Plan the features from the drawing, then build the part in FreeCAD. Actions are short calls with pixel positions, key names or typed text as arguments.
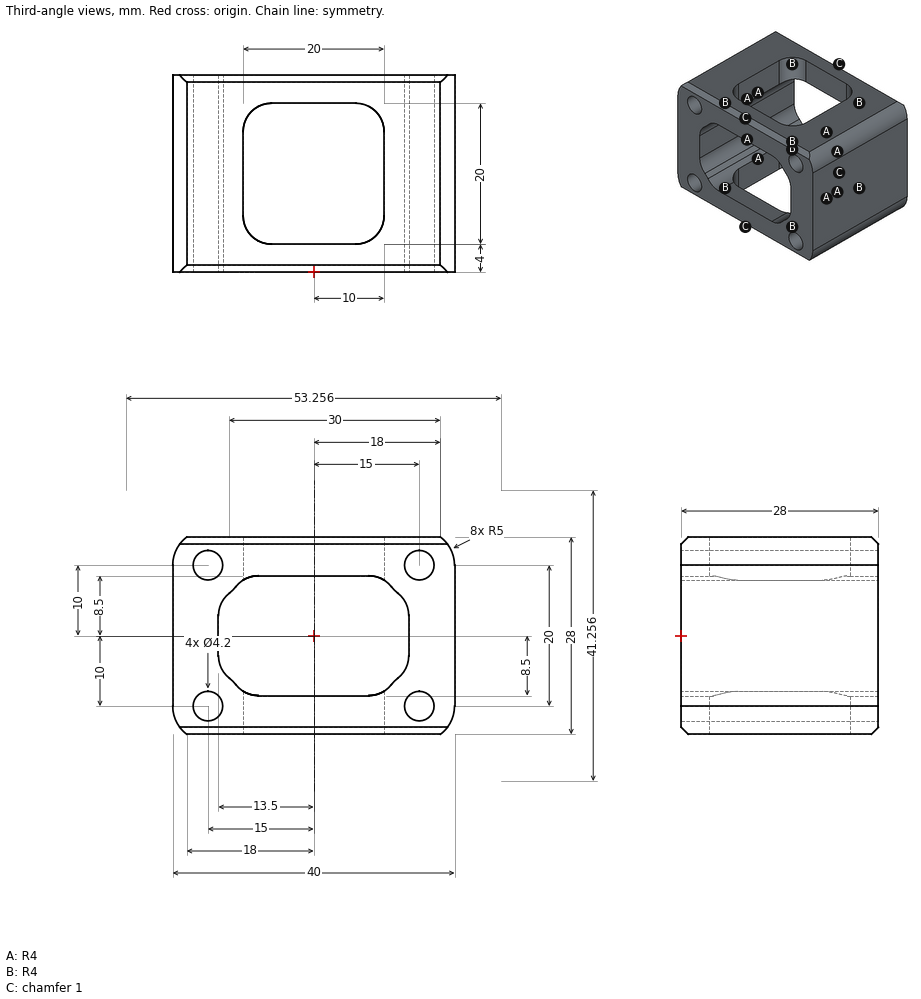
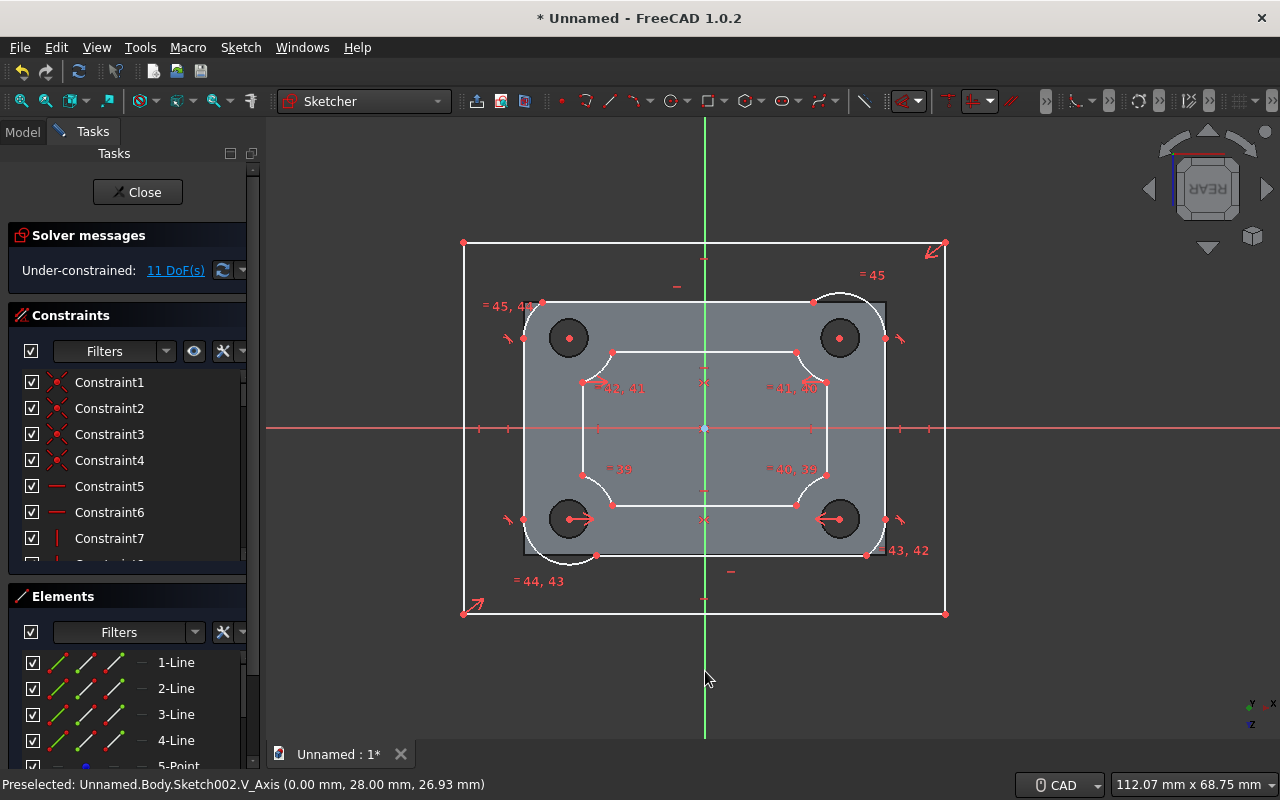
click(607, 494)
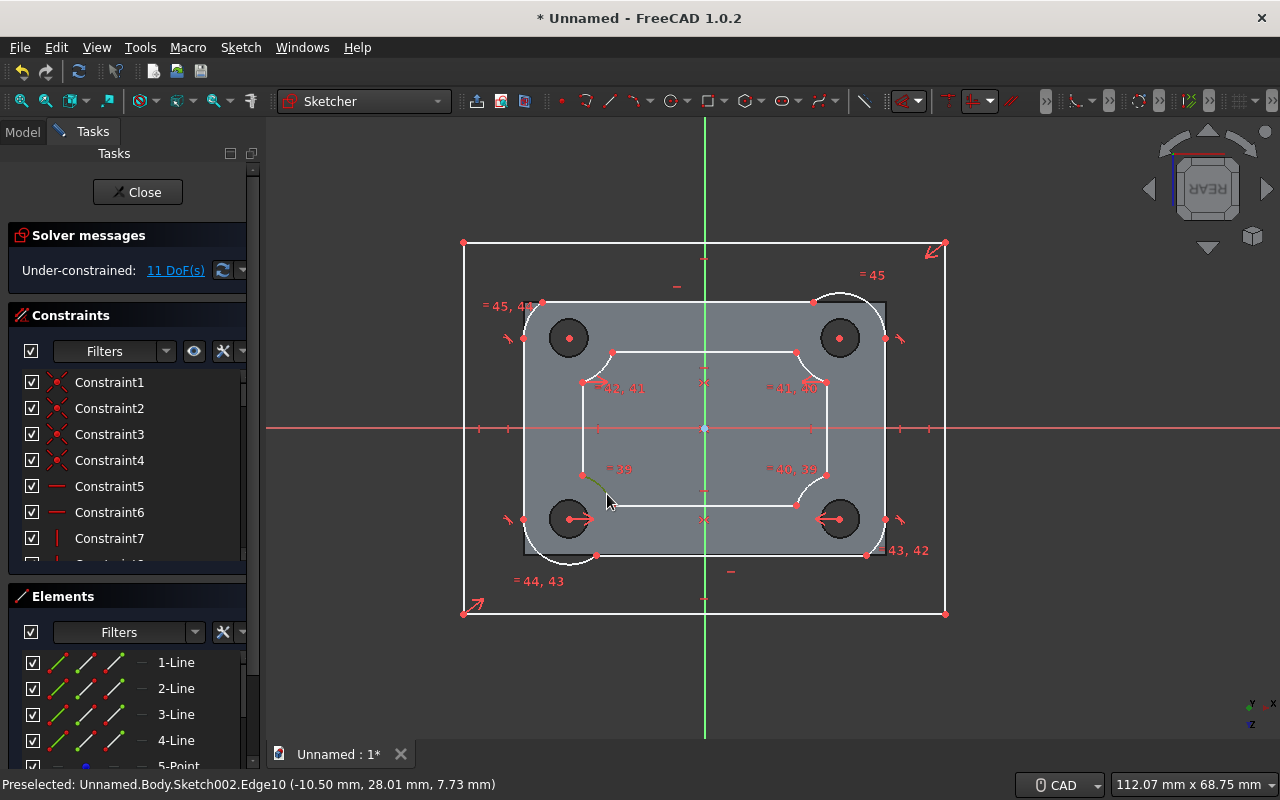
click(920, 102)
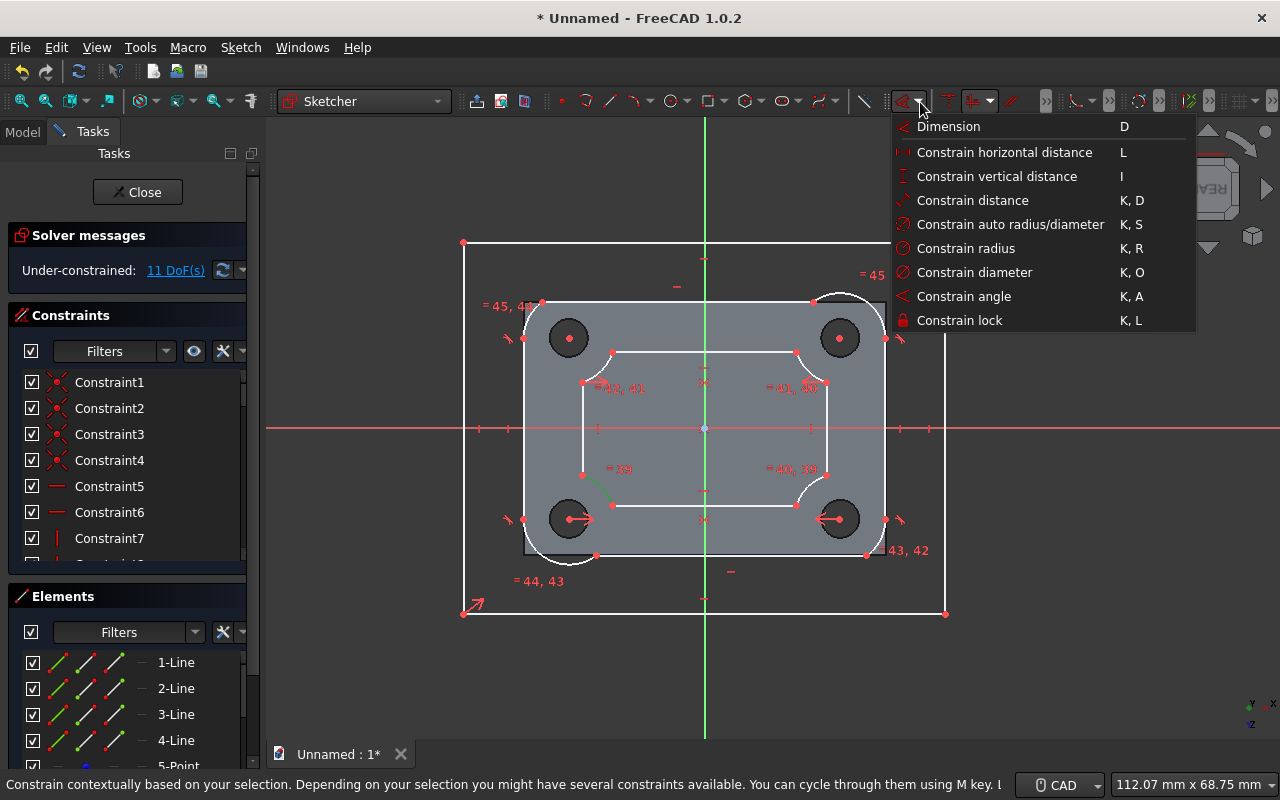
click(1044, 248)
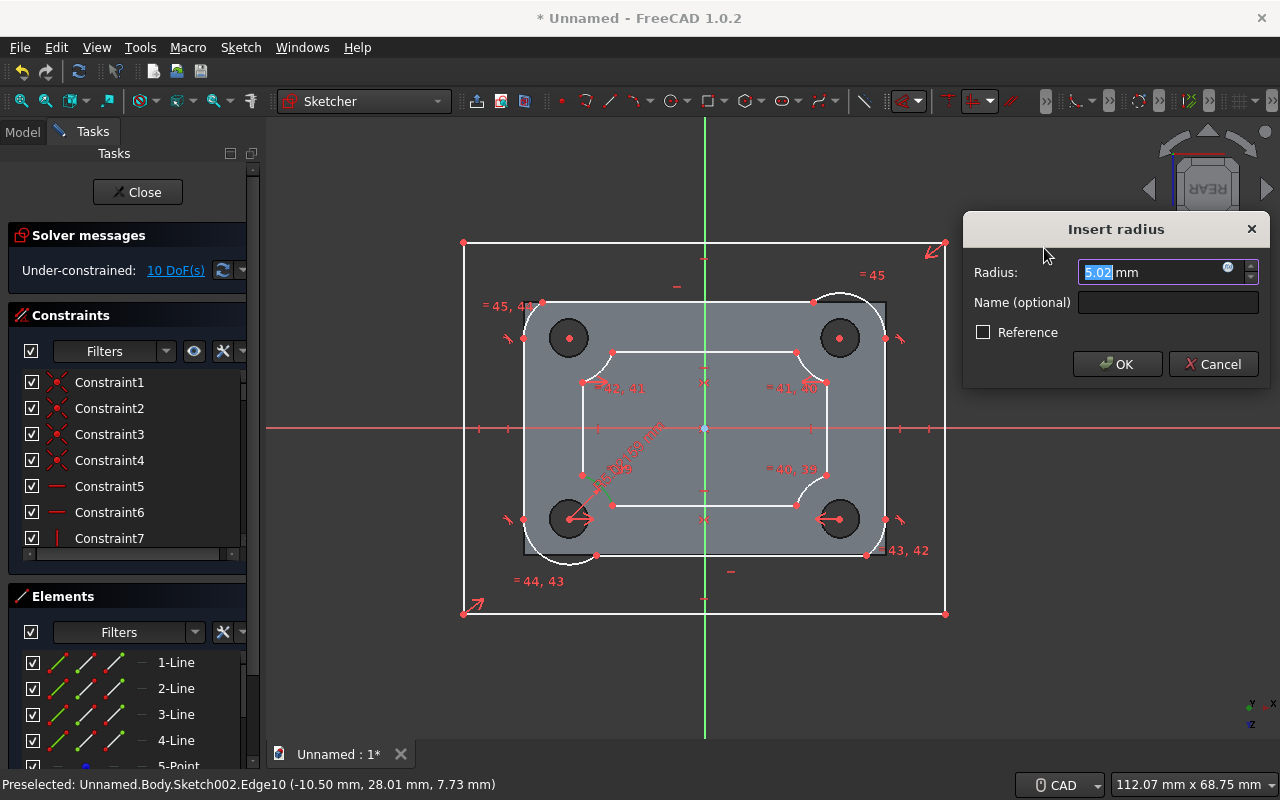
text(5)
key(Return)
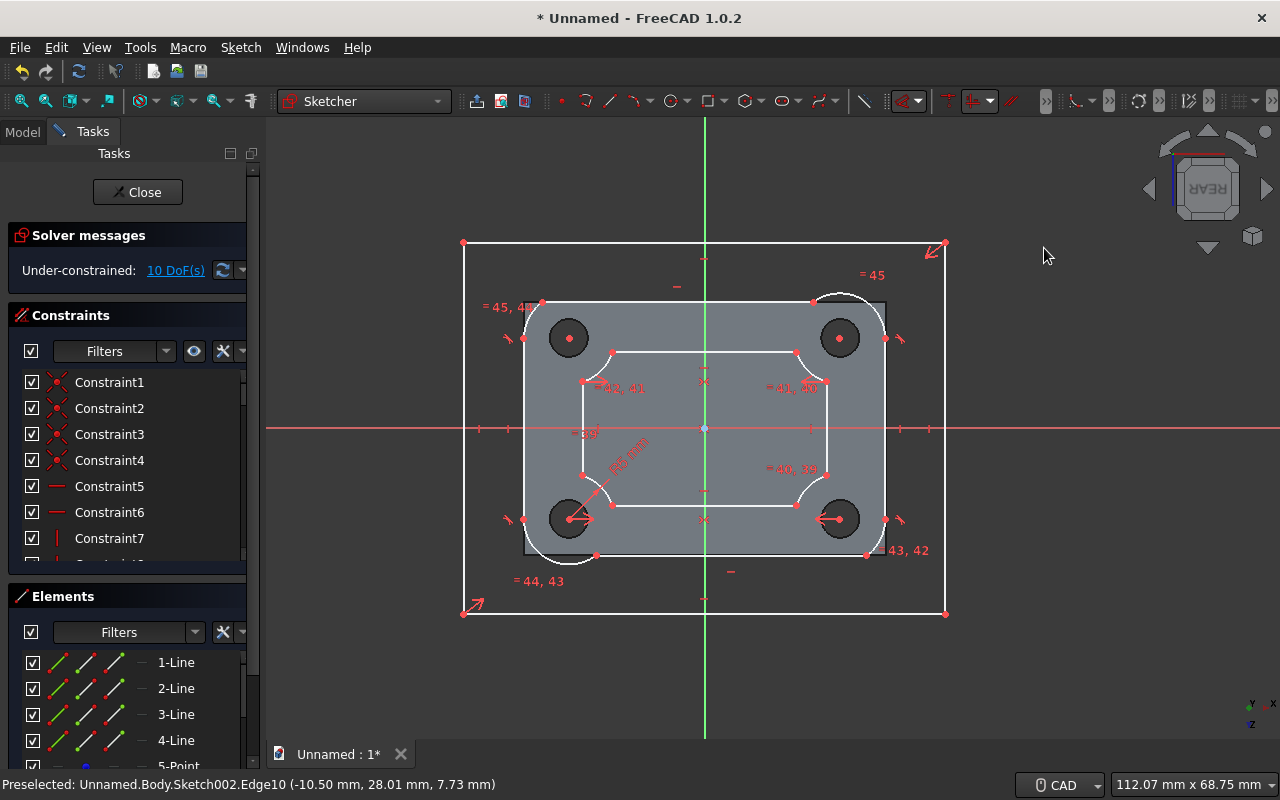
click(885, 393)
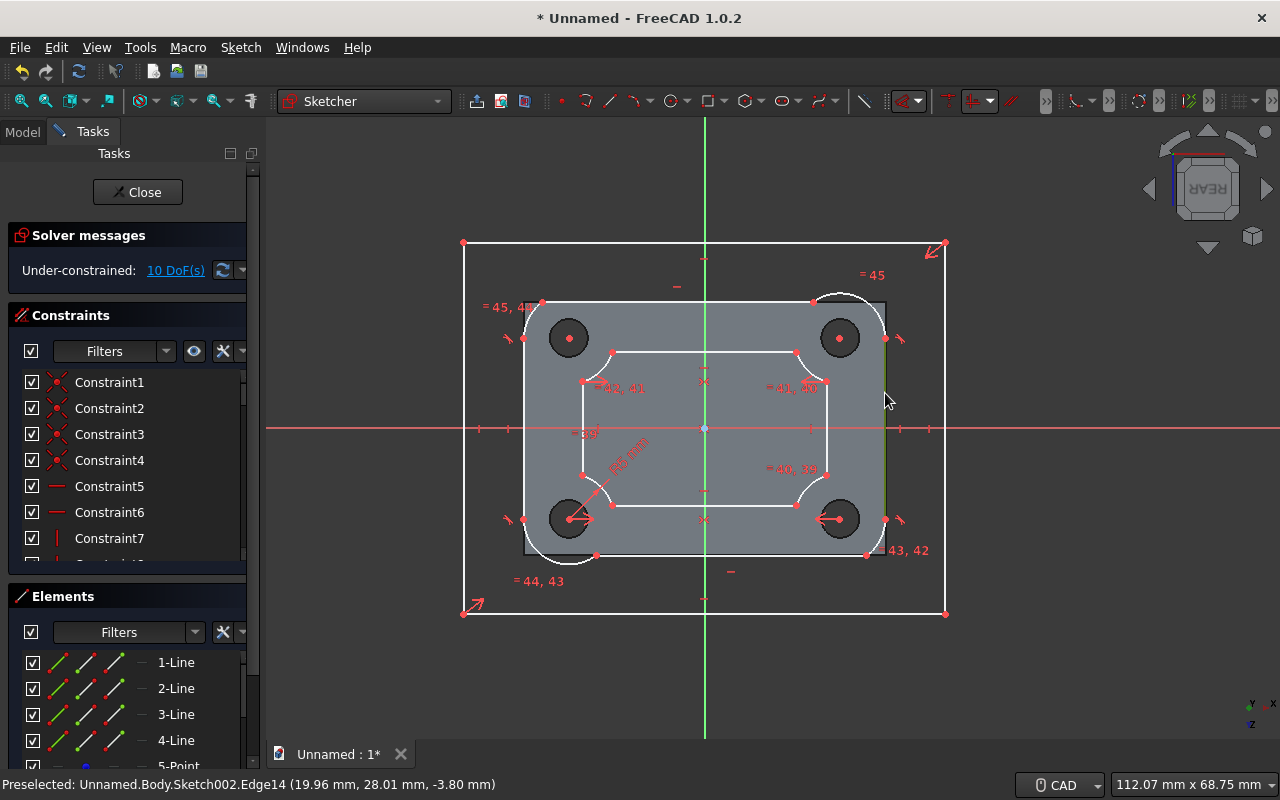
key(i)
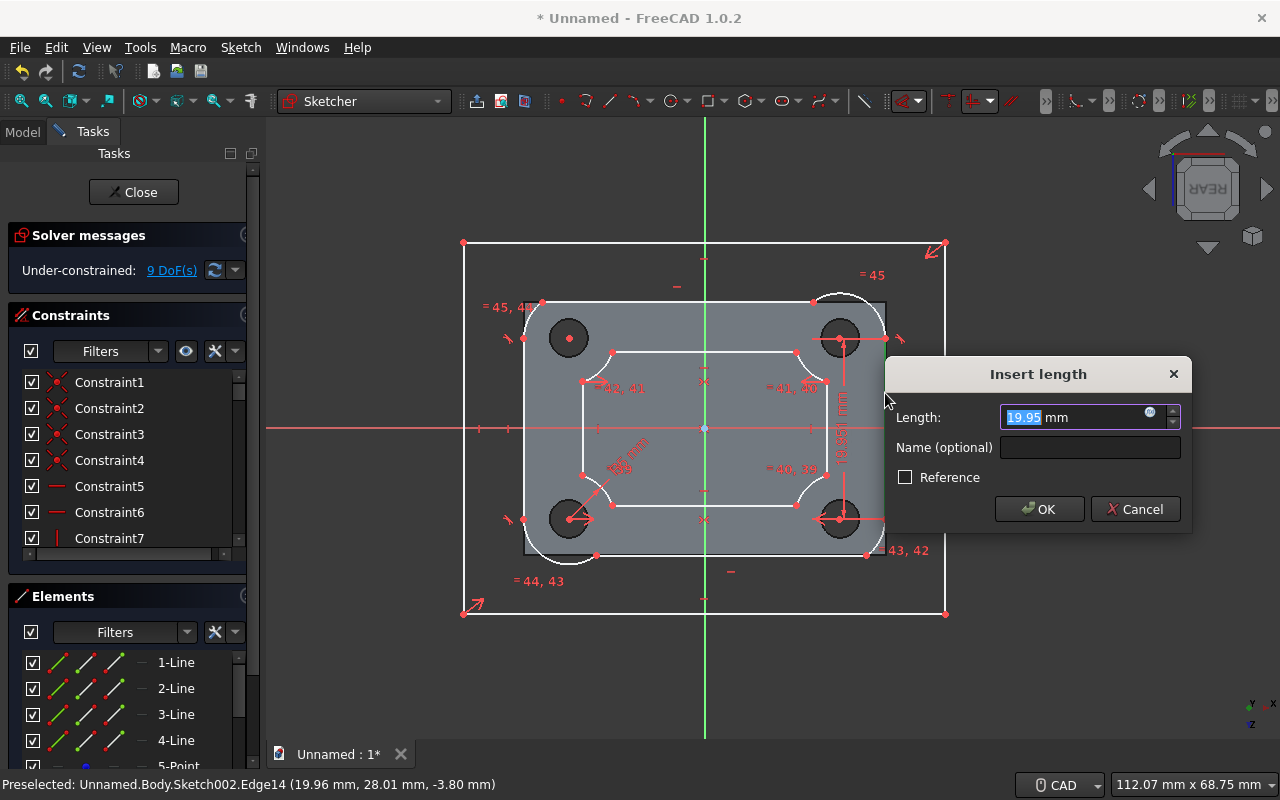
text(20)
key(Return)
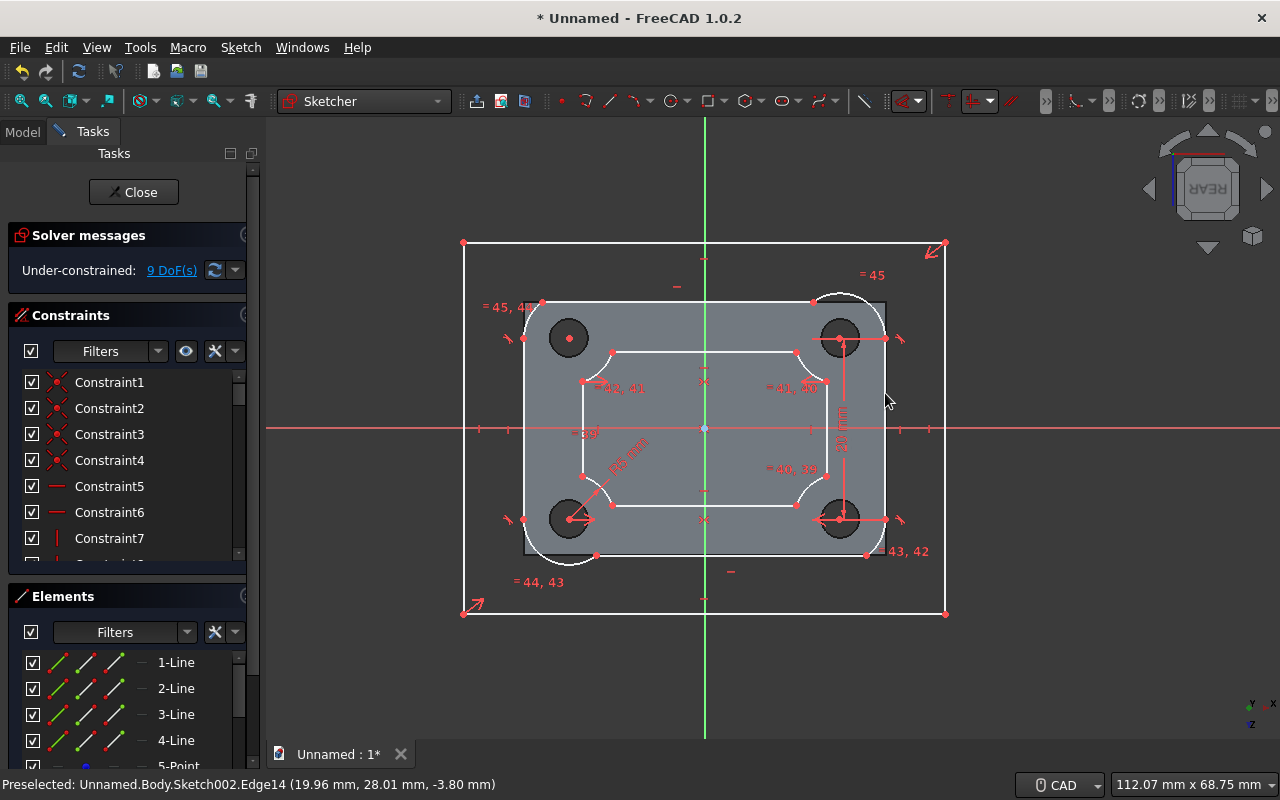
click(786, 556)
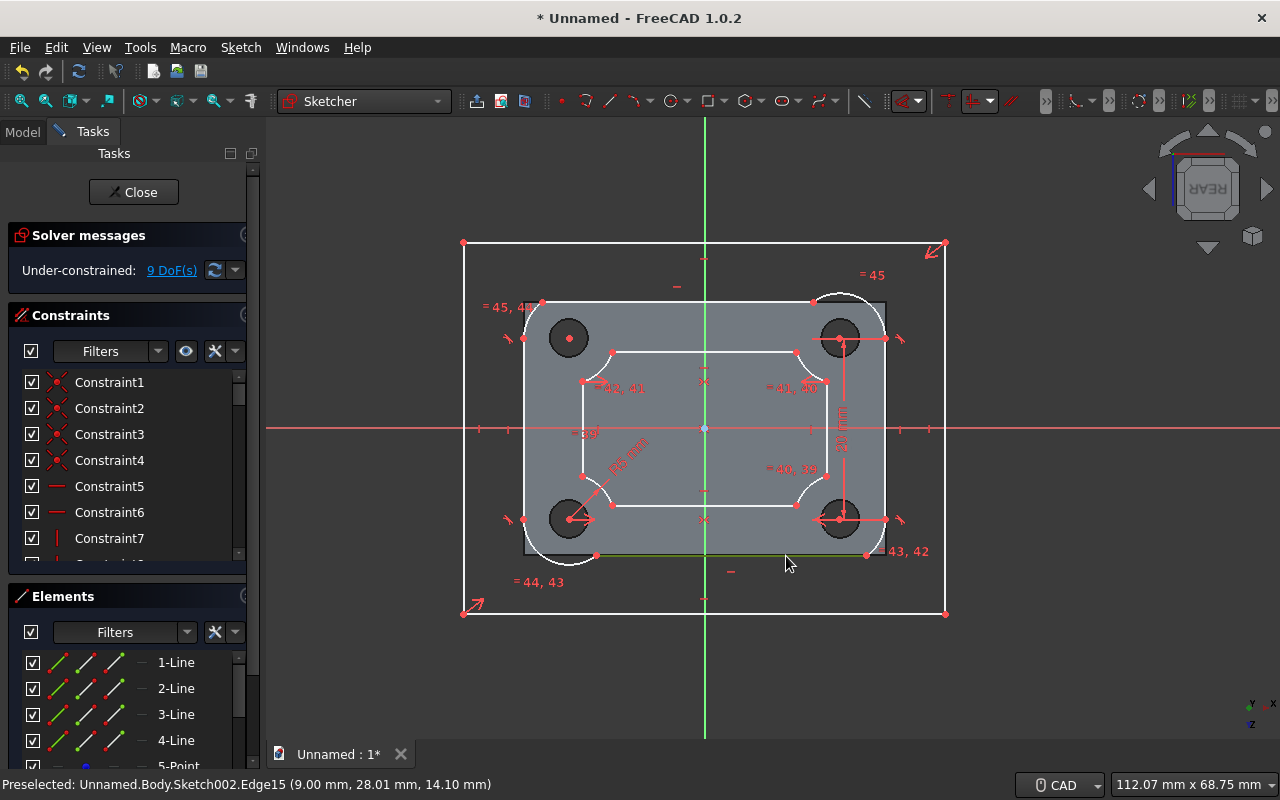
key(l)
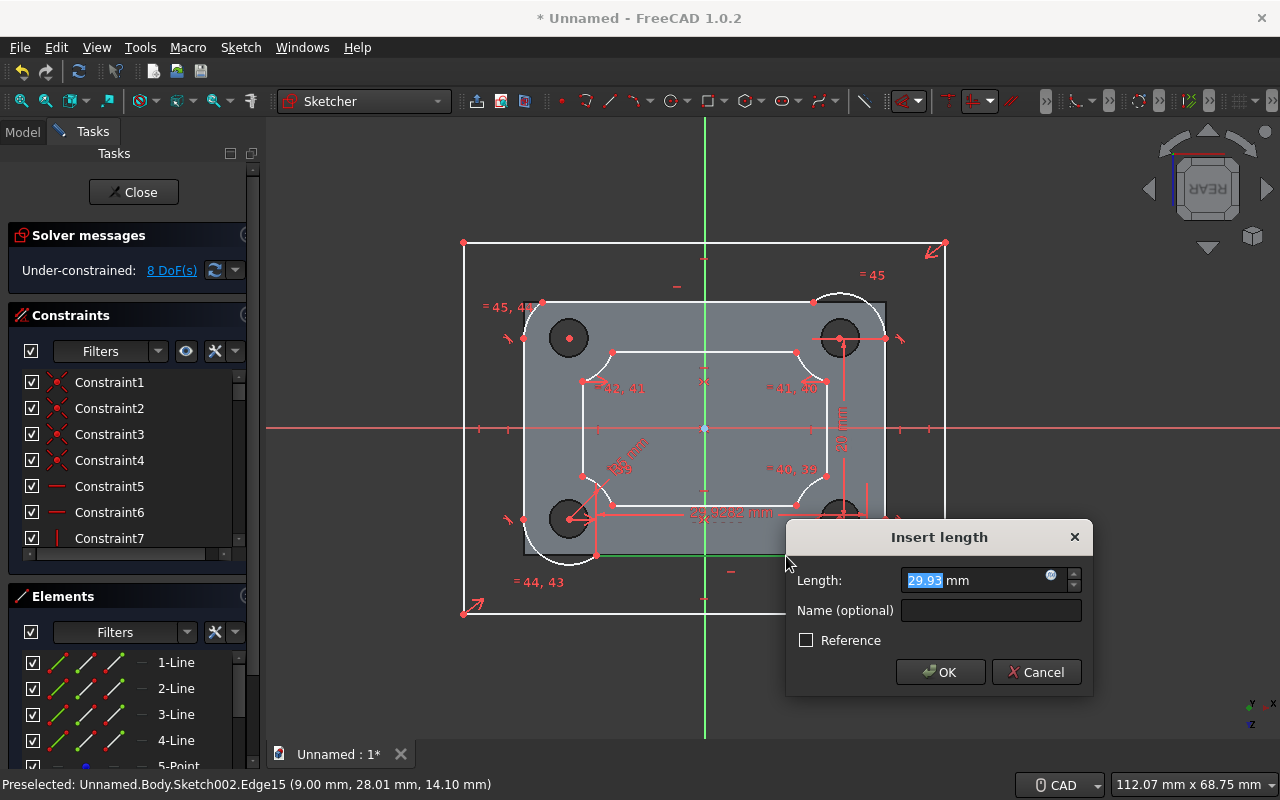
text(30)
key(Return)